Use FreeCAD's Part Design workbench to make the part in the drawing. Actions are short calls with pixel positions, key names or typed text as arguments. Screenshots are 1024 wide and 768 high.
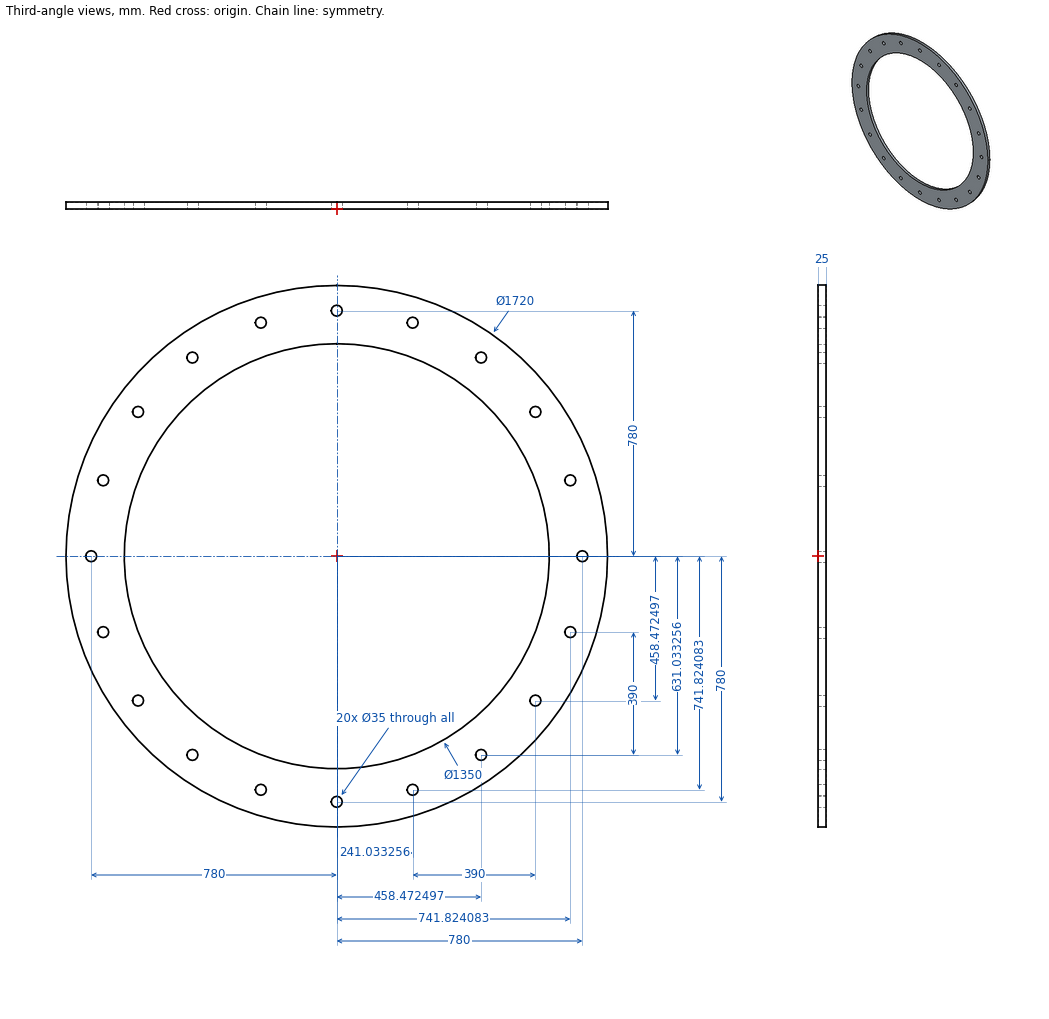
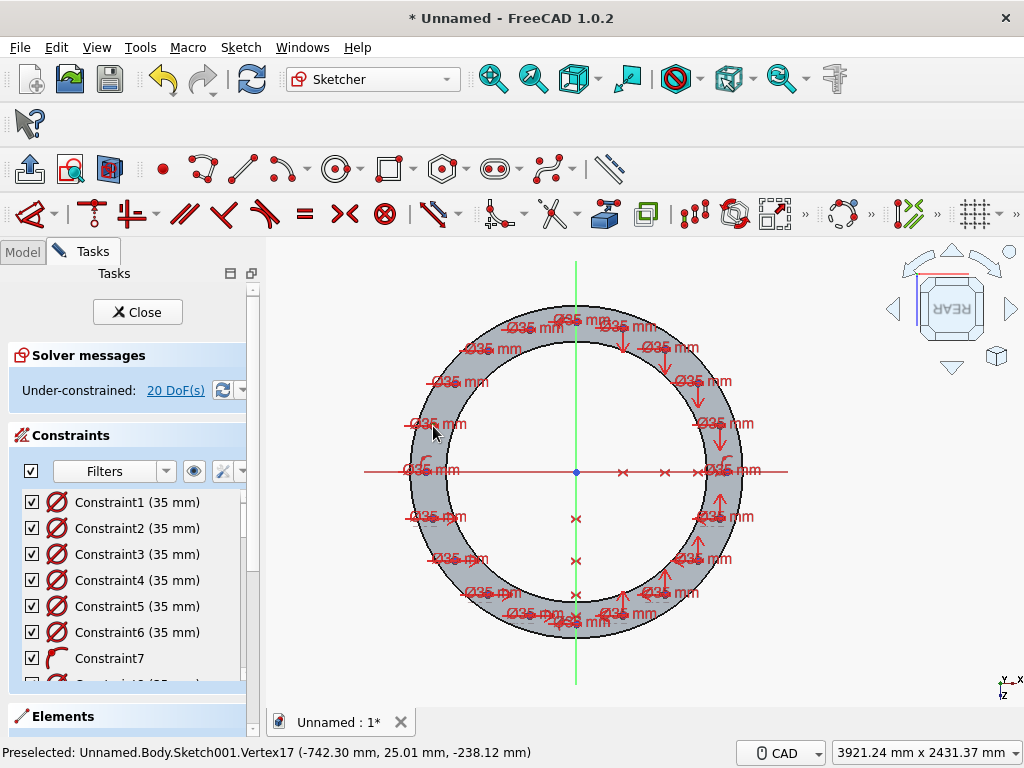
click(576, 531)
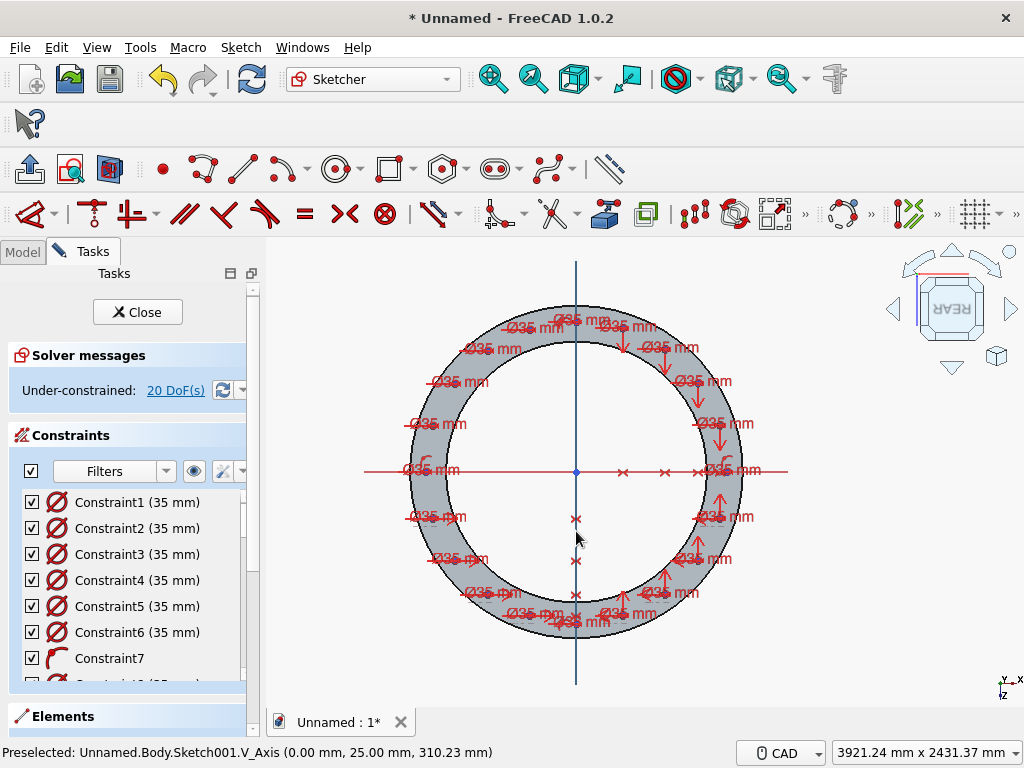
key(s)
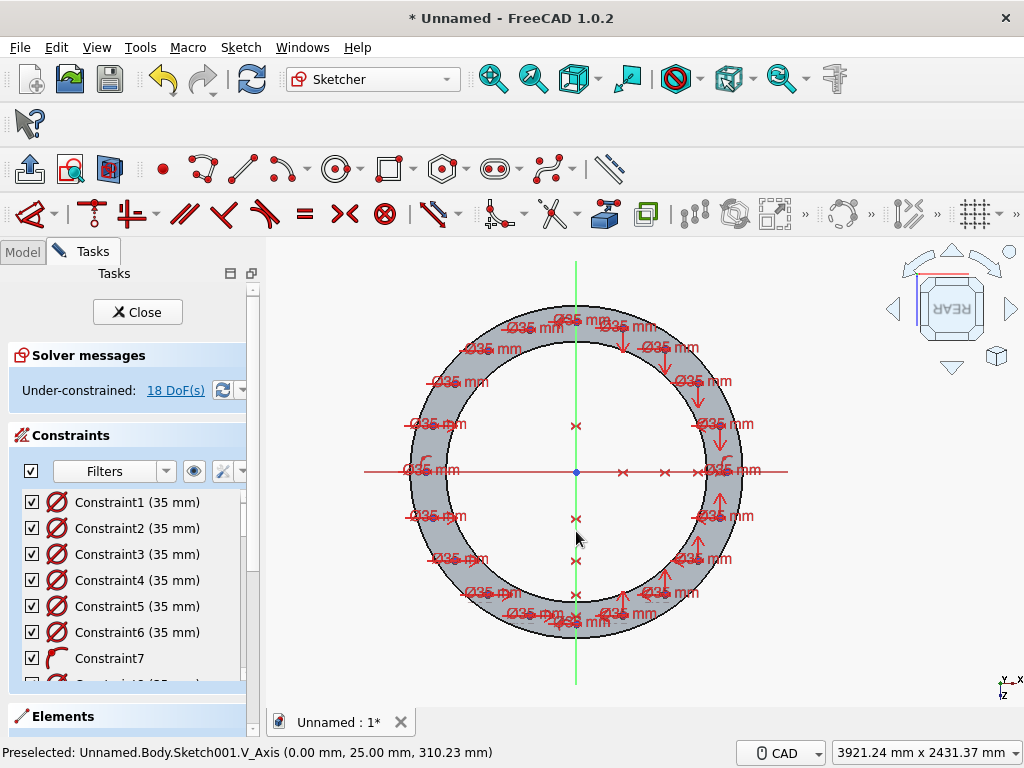
click(698, 383)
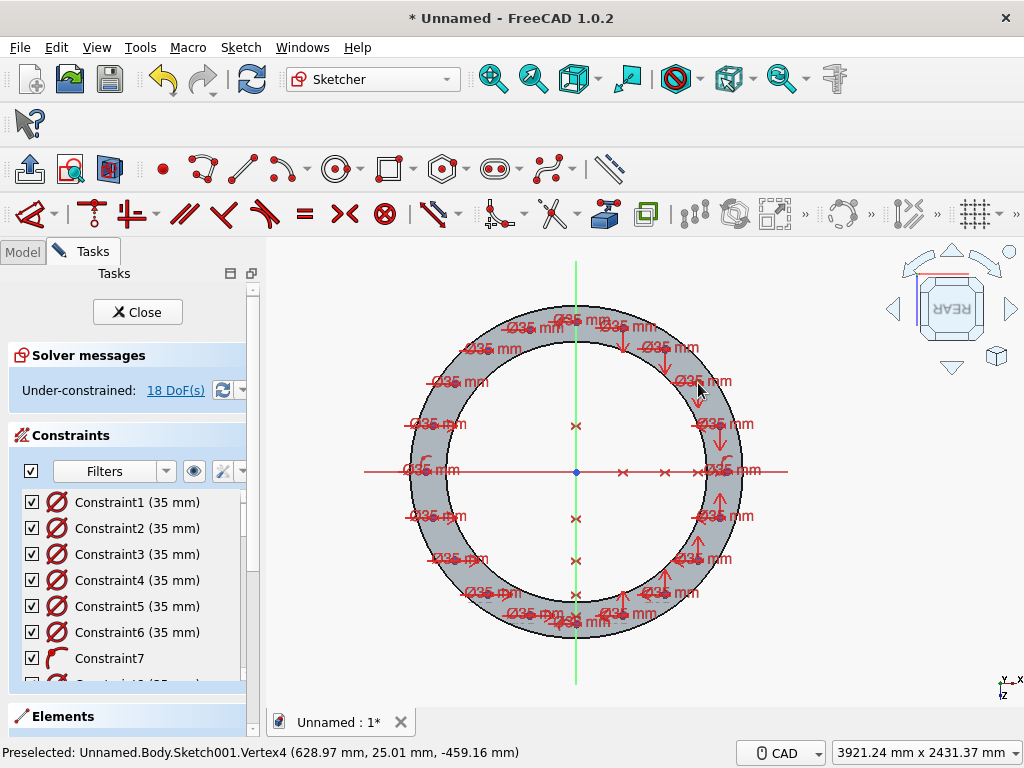
click(455, 384)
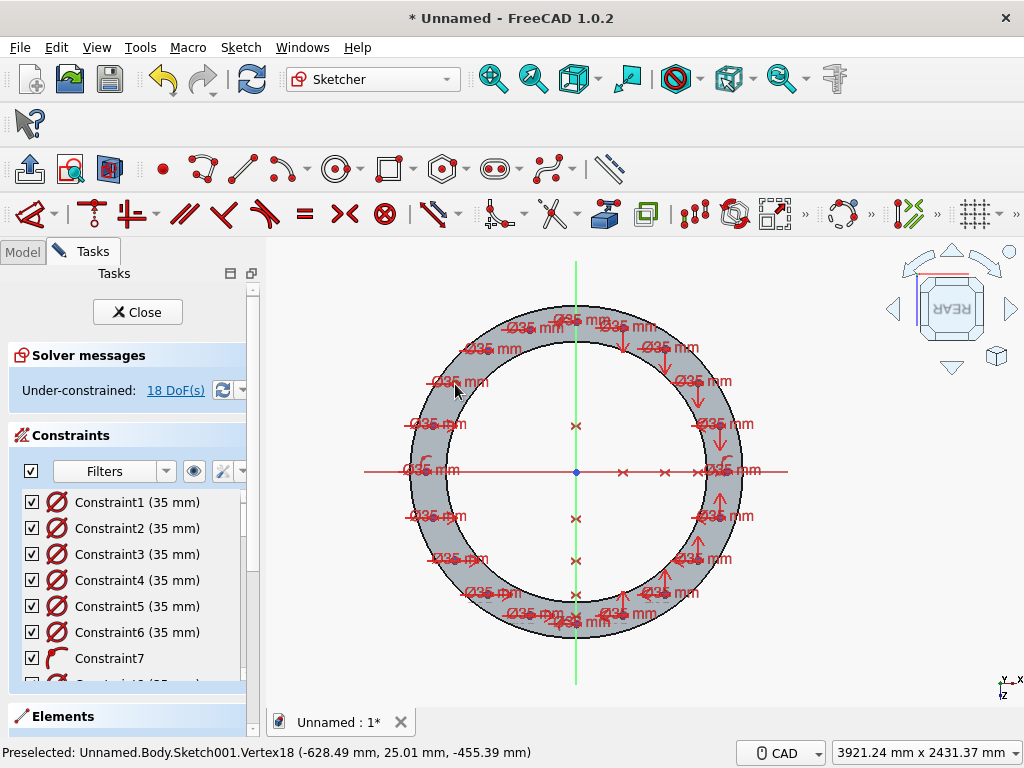
click(576, 531)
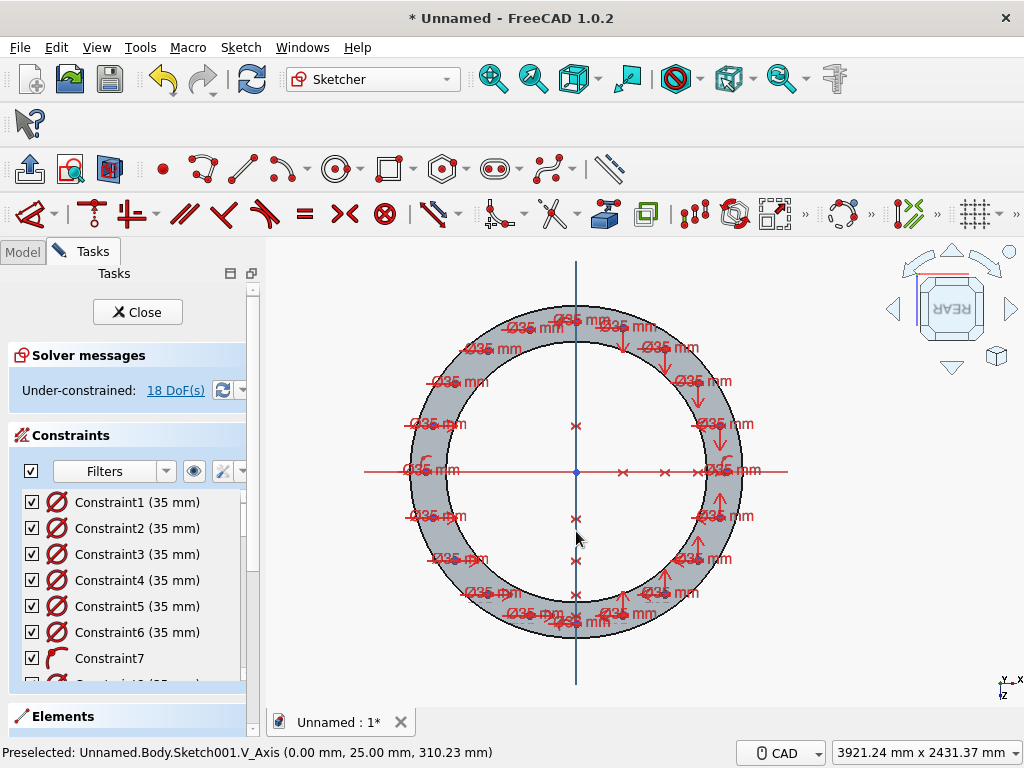
key(s)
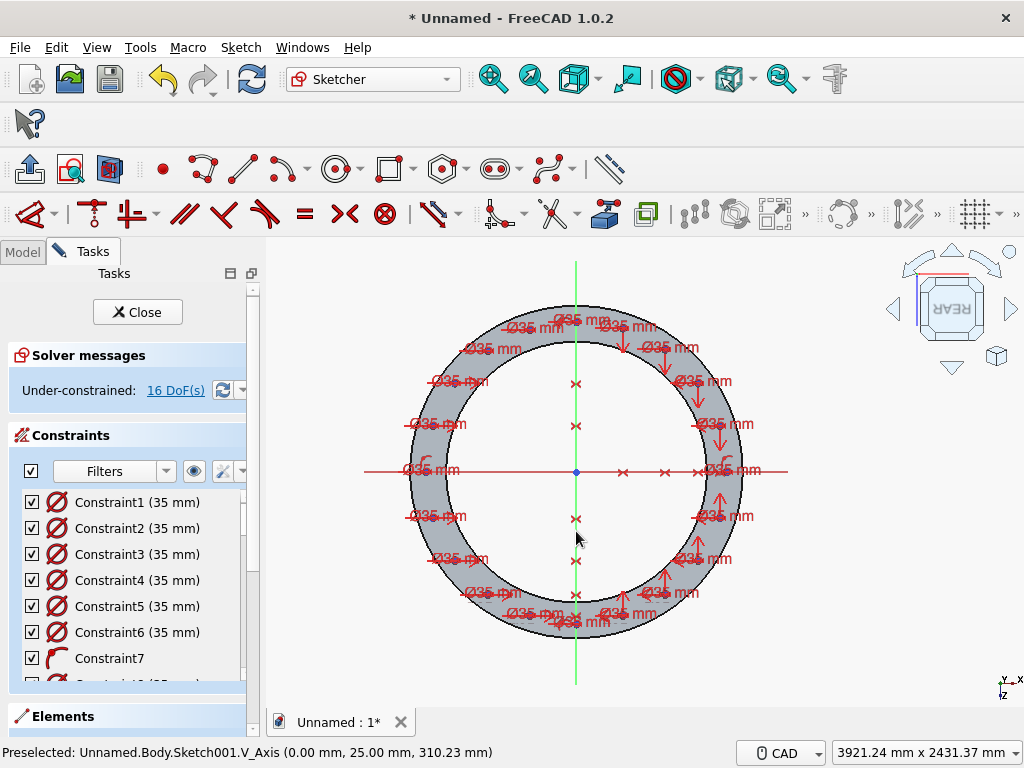
click(665, 349)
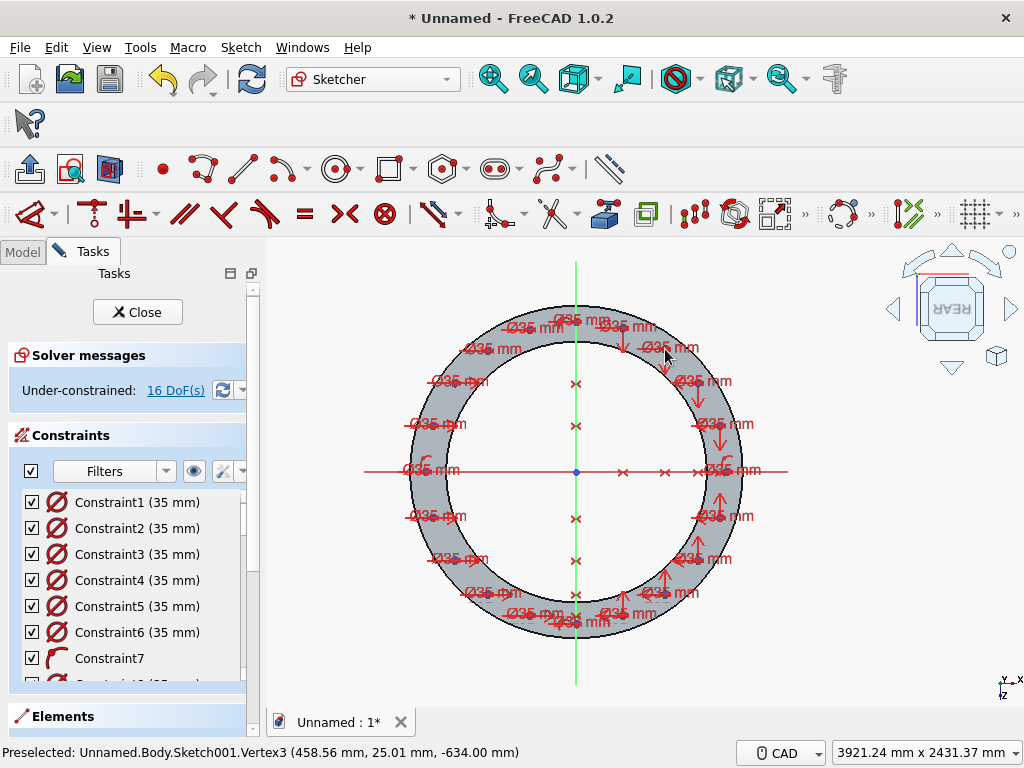
click(488, 351)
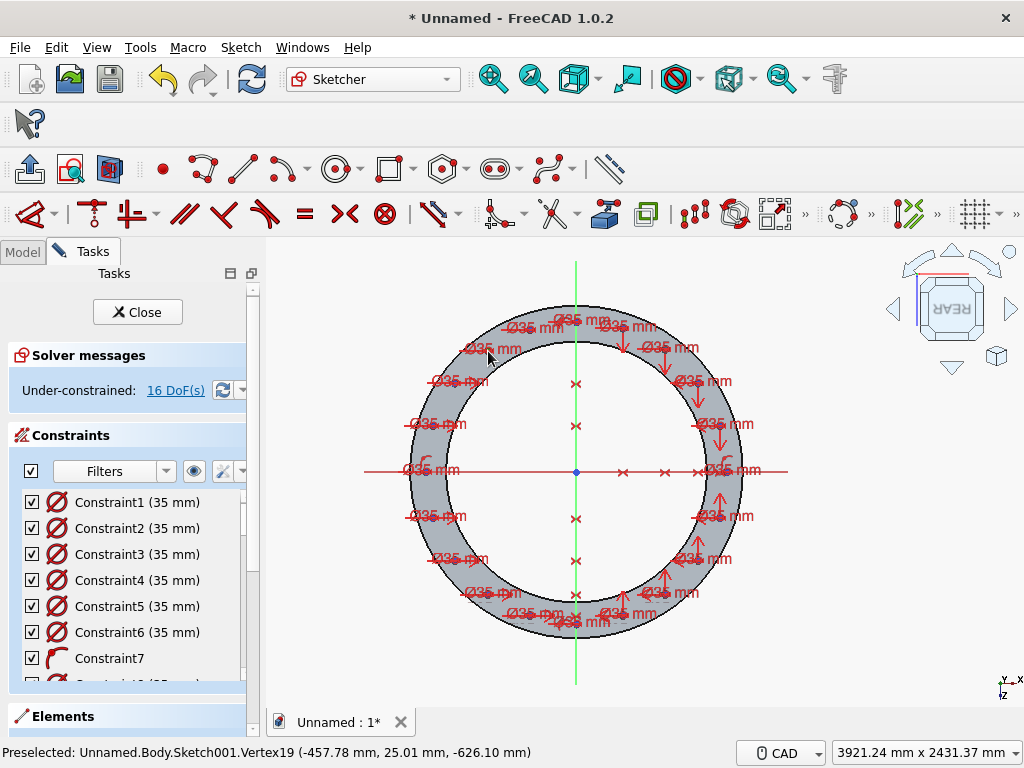
click(576, 531)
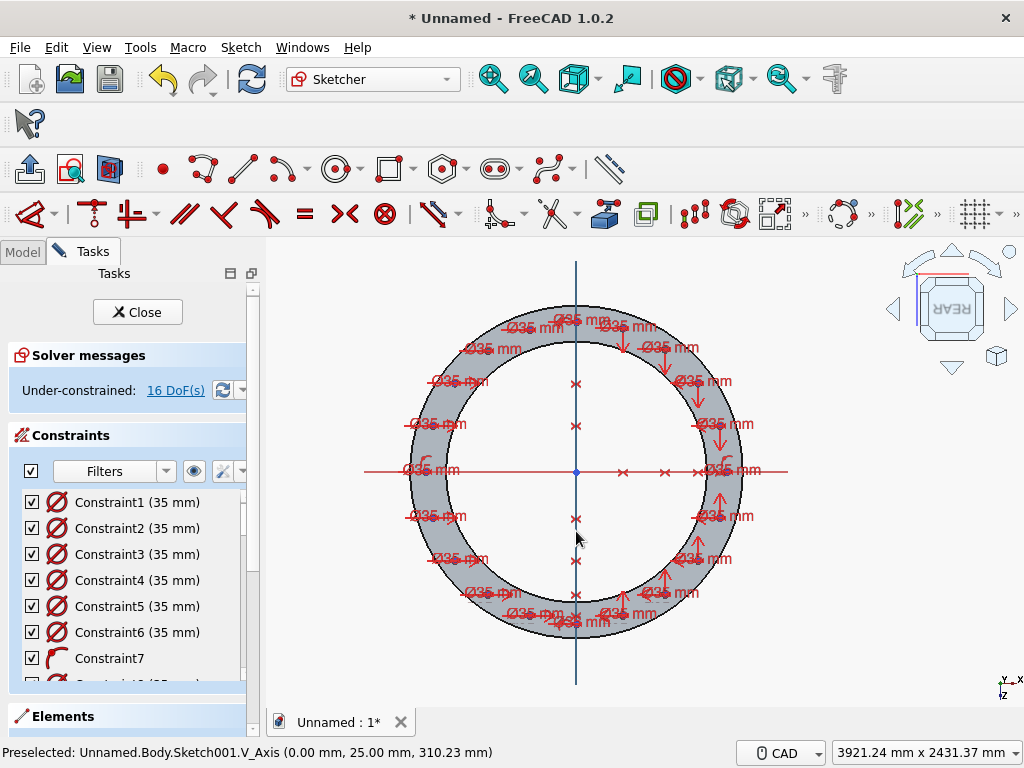
click(346, 214)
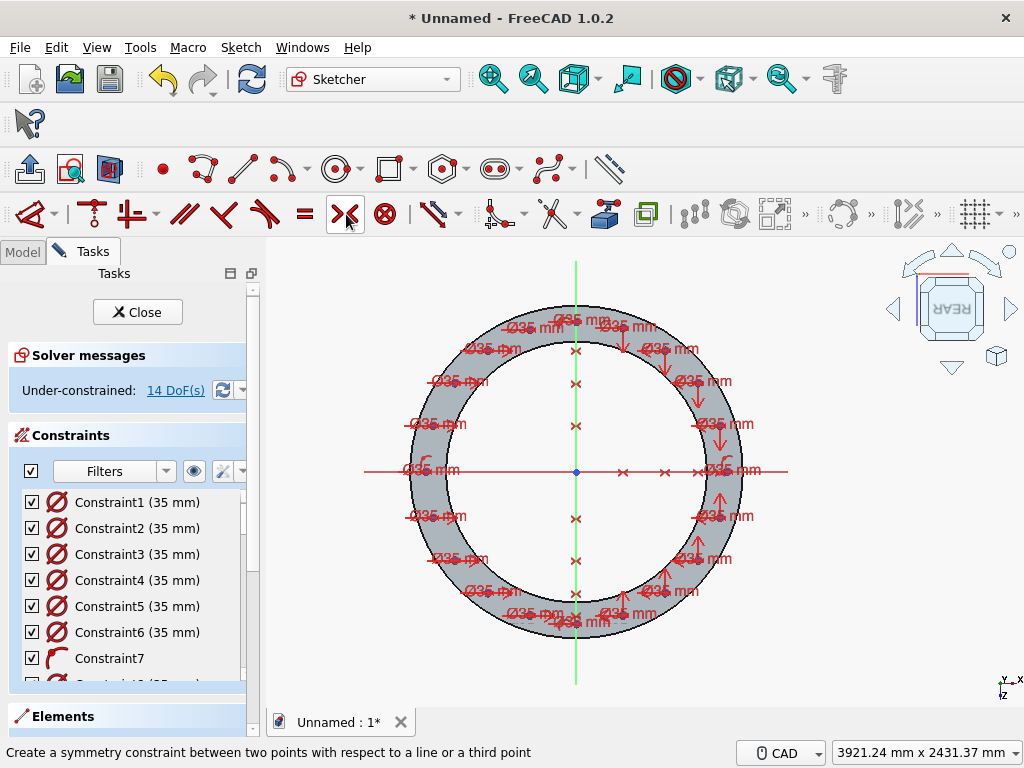
click(623, 328)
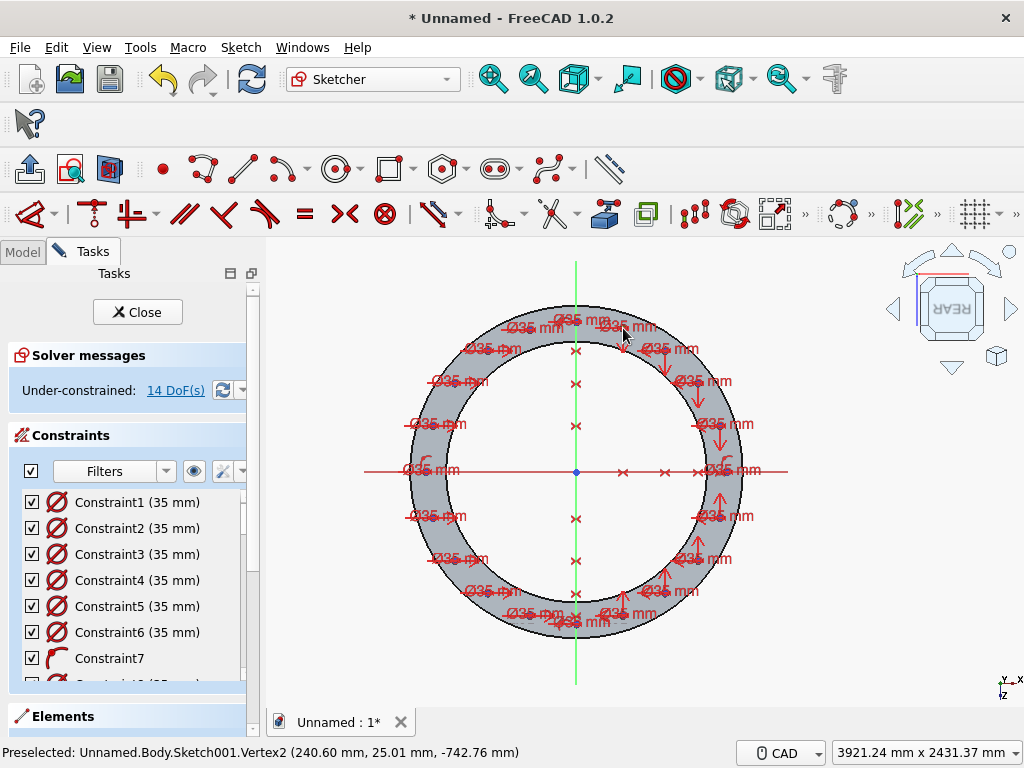
click(530, 330)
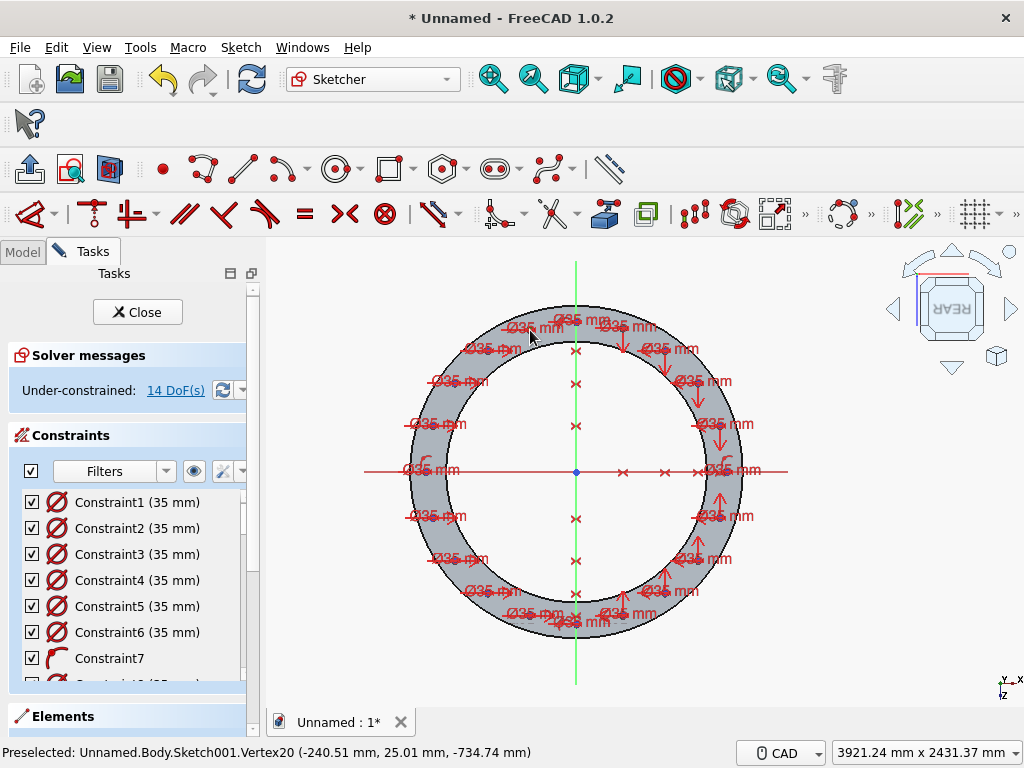
click(576, 531)